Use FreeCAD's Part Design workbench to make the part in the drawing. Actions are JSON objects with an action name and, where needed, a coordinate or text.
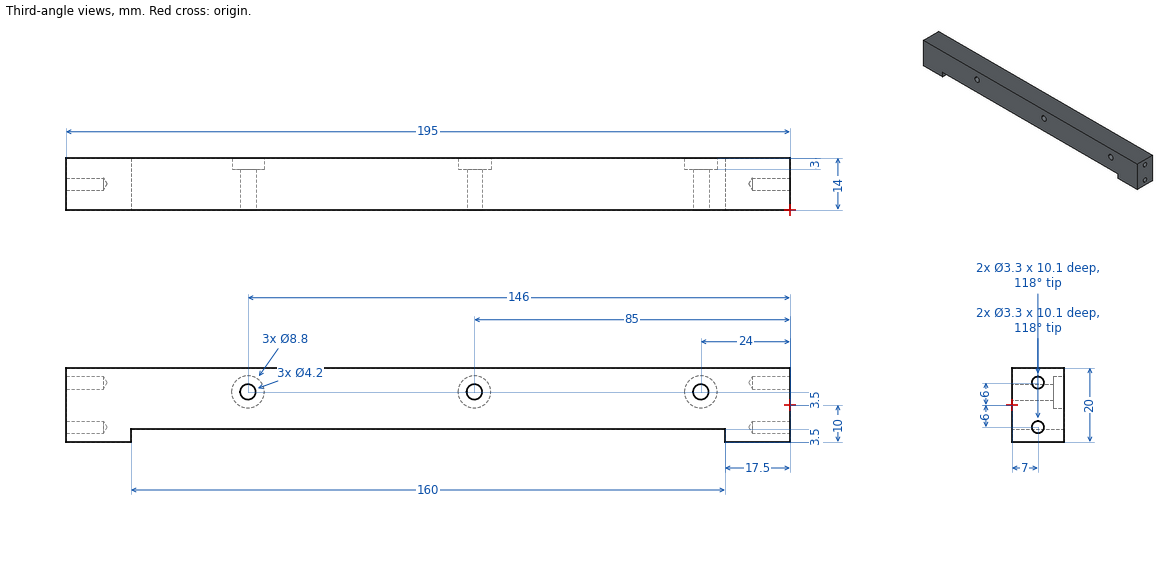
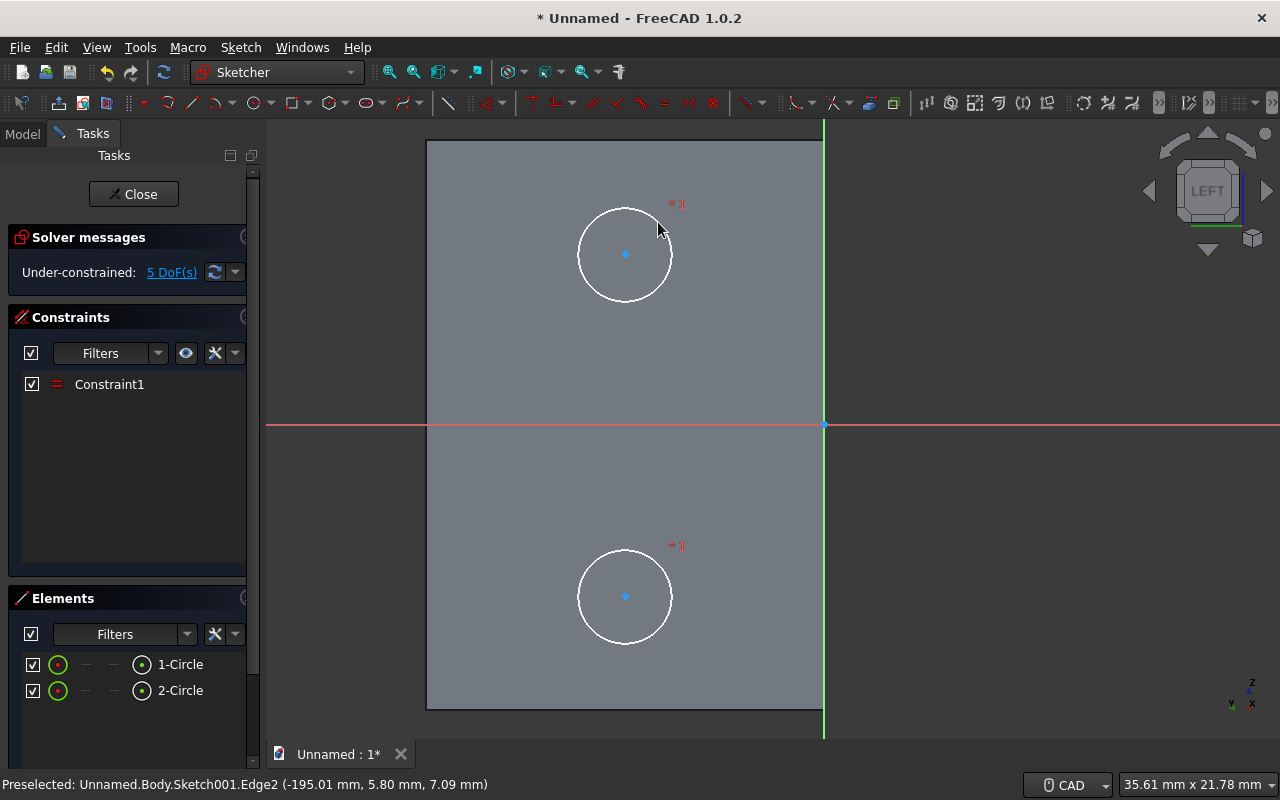
{"action": "left_click", "coordinate": [658, 564]}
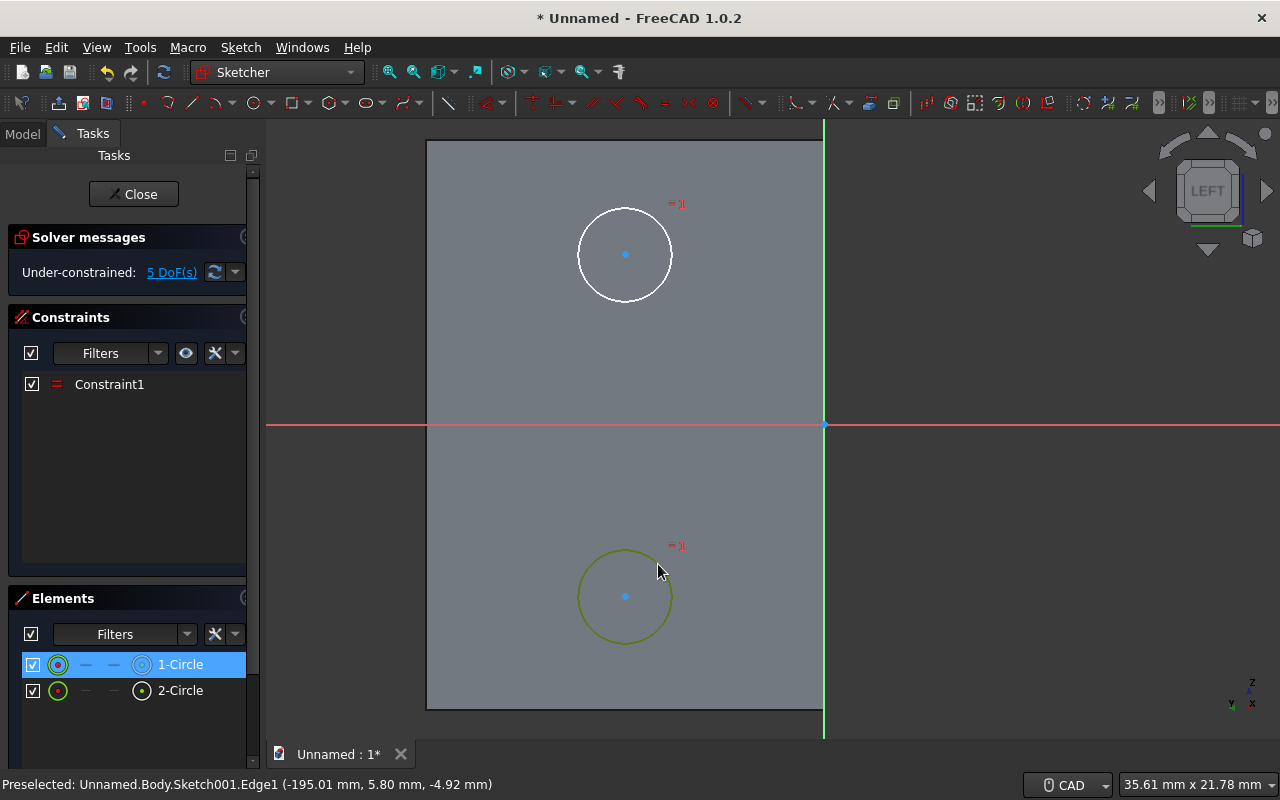
{"action": "key", "text": "k o"}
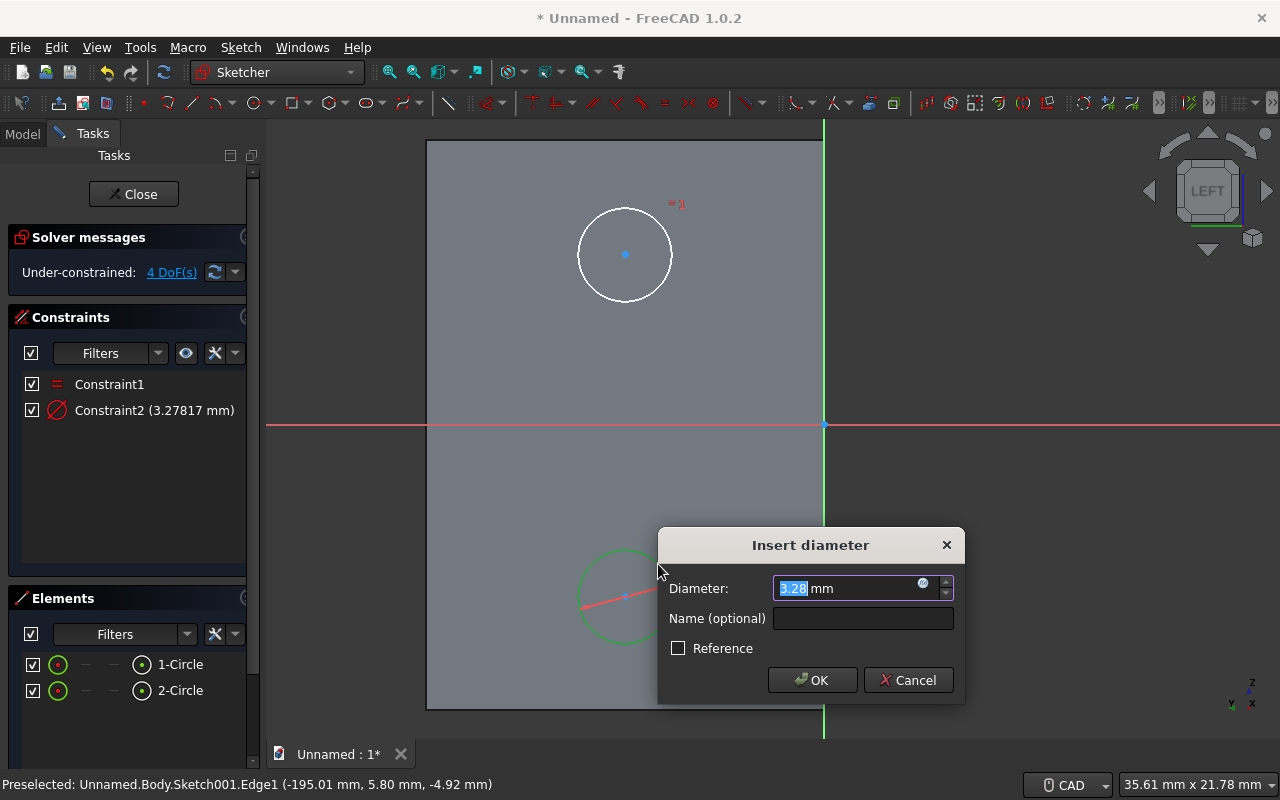
{"action": "type", "text": "3.3"}
{"action": "key", "text": "Return"}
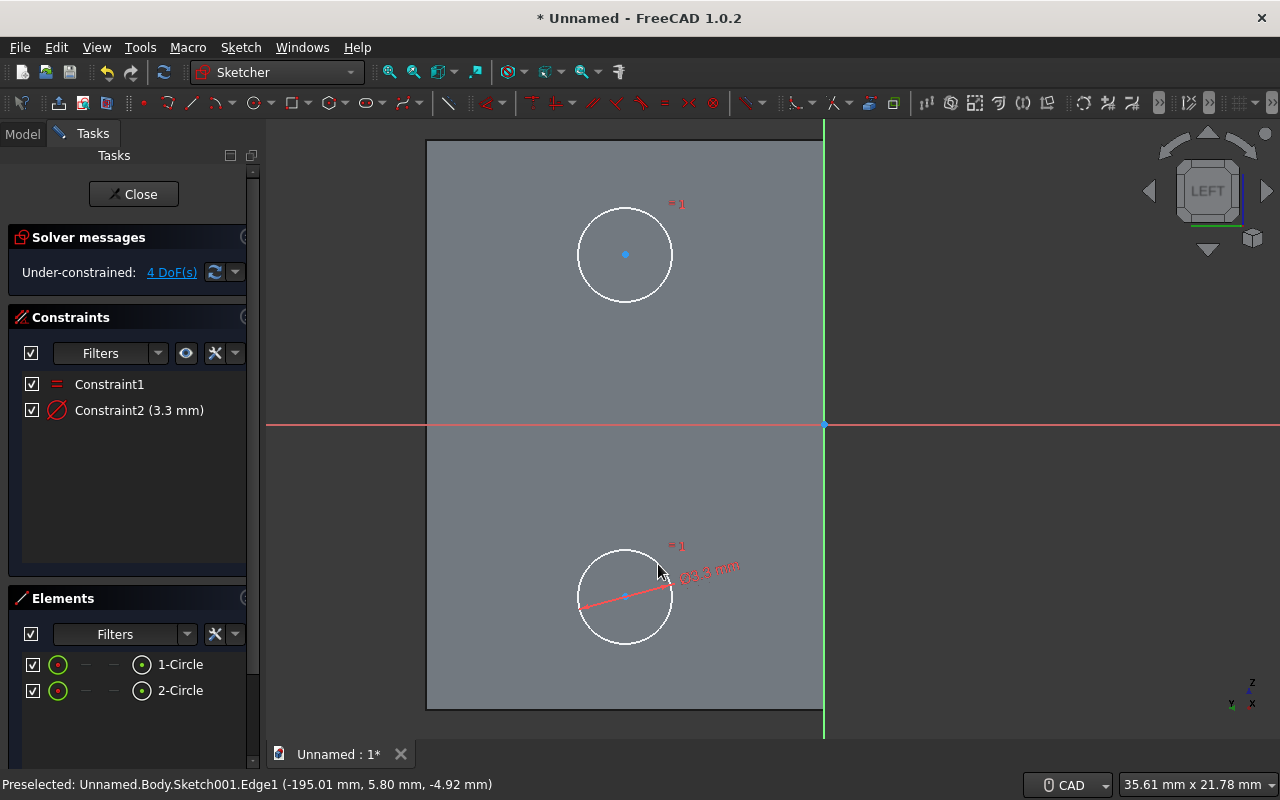
{"action": "left_click", "coordinate": [625, 597]}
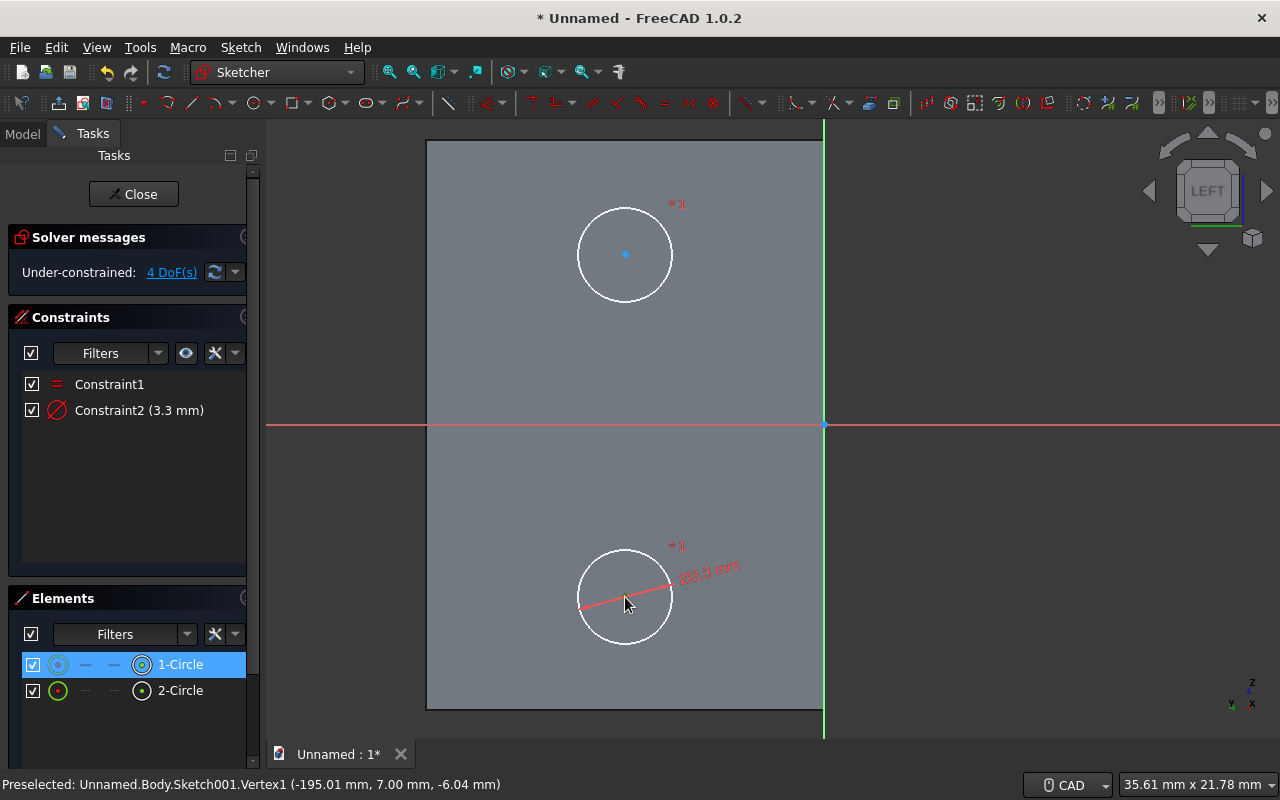
{"action": "key", "text": "l"}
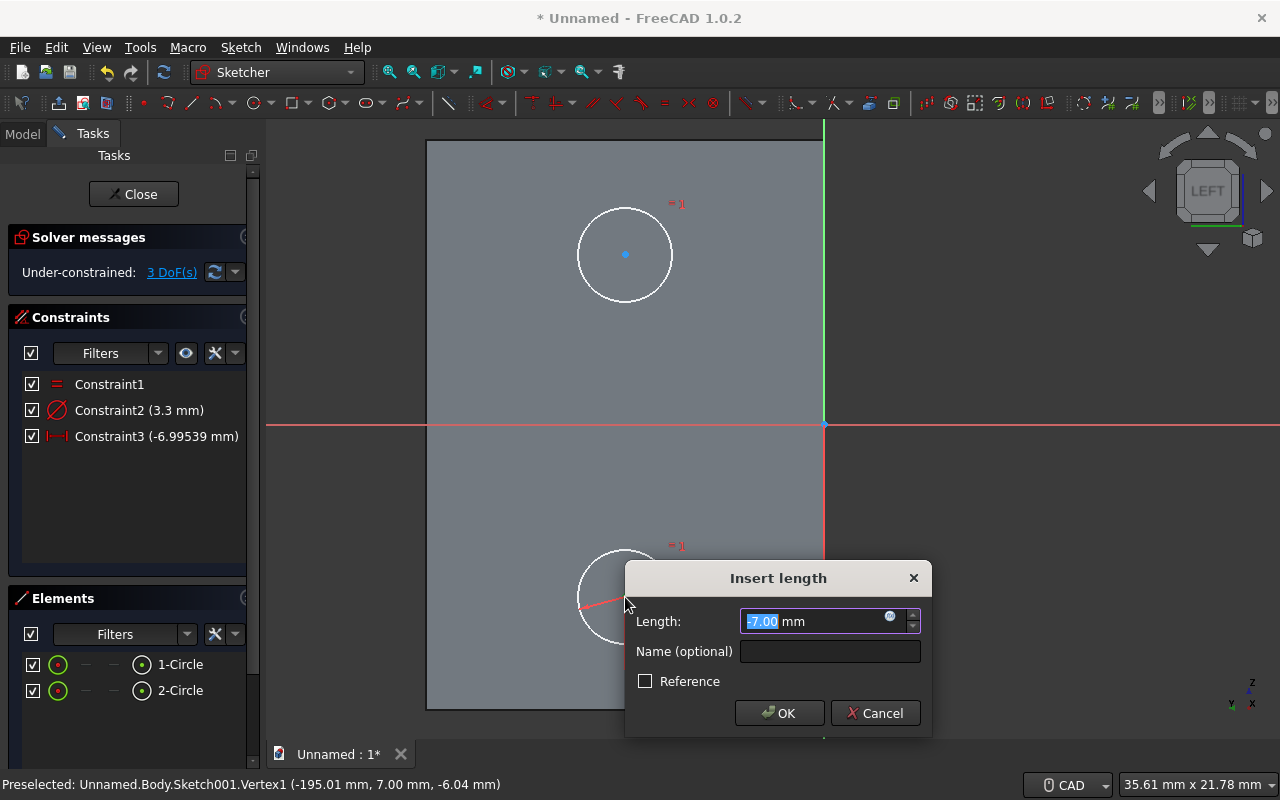
{"action": "type", "text": "-7"}
{"action": "key", "text": "Return"}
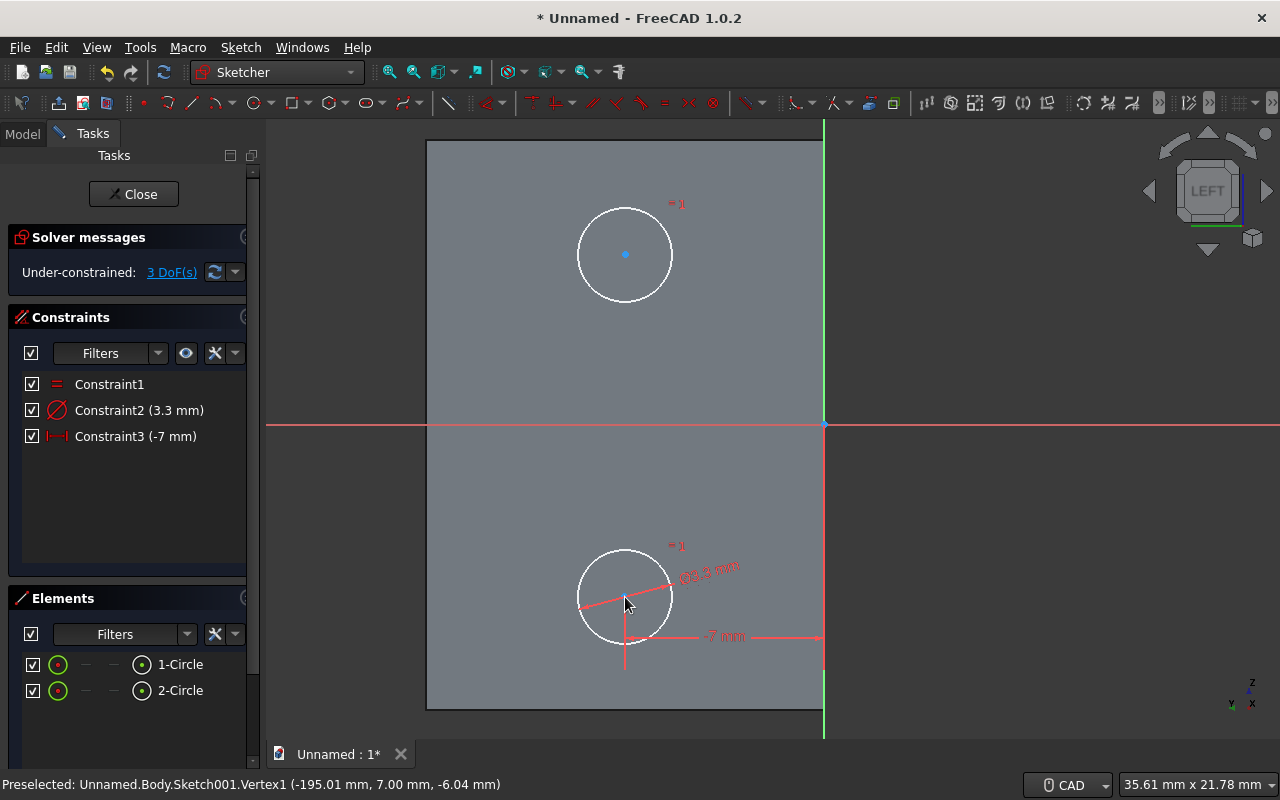
{"action": "left_click", "coordinate": [625, 597]}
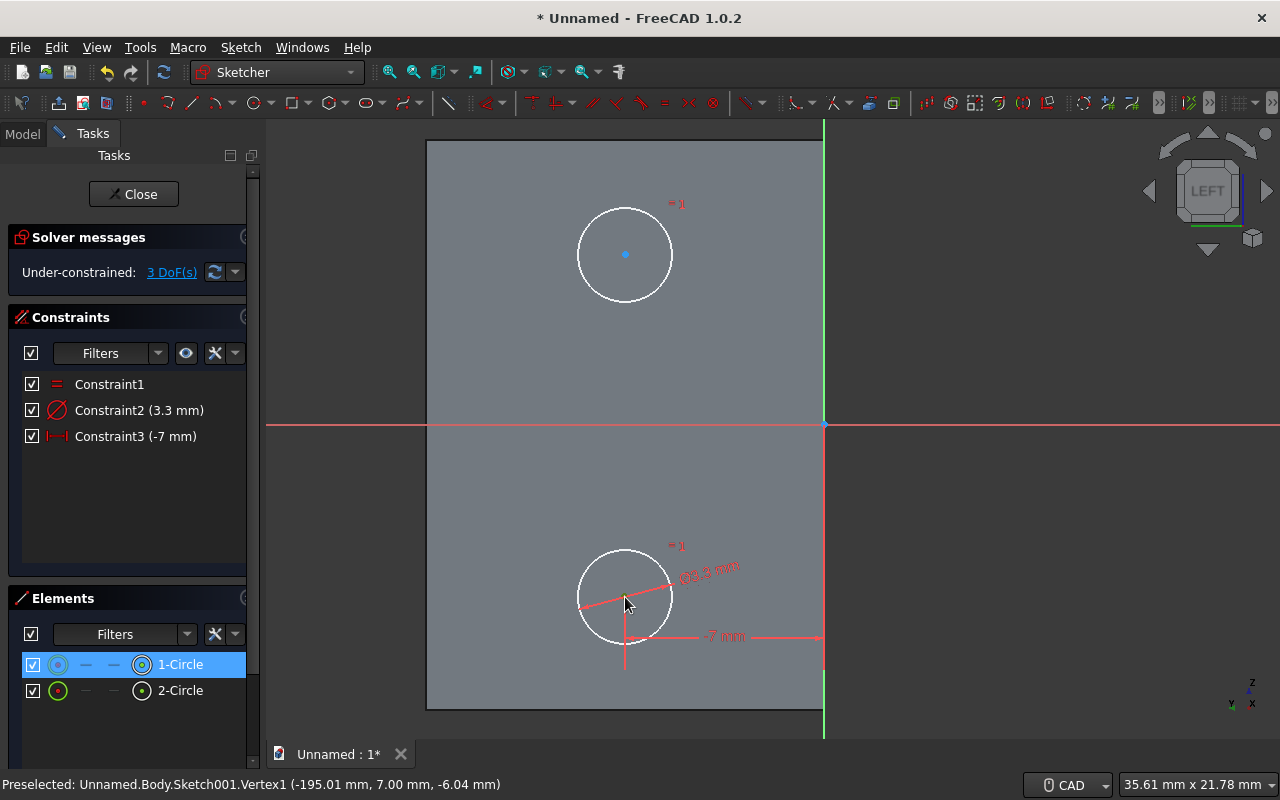
{"action": "left_click", "coordinate": [504, 104]}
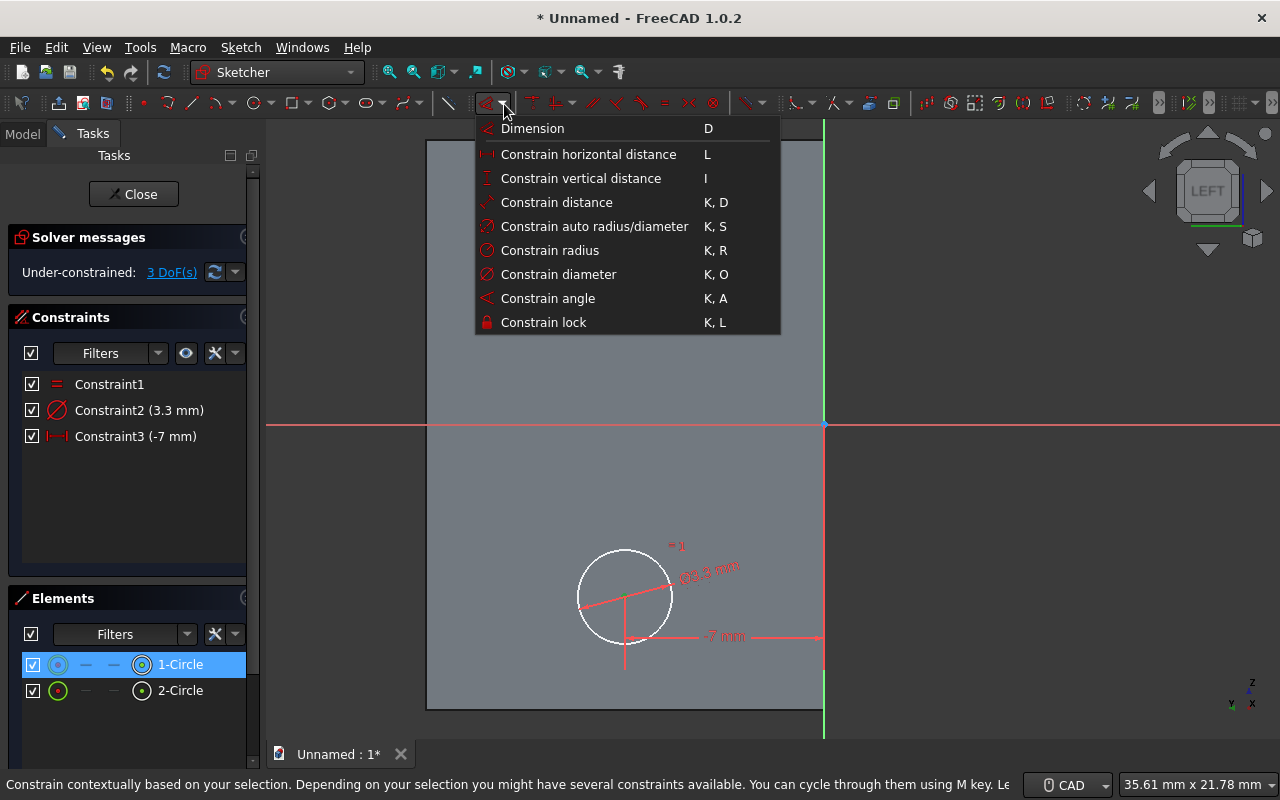
{"action": "left_click", "coordinate": [628, 178]}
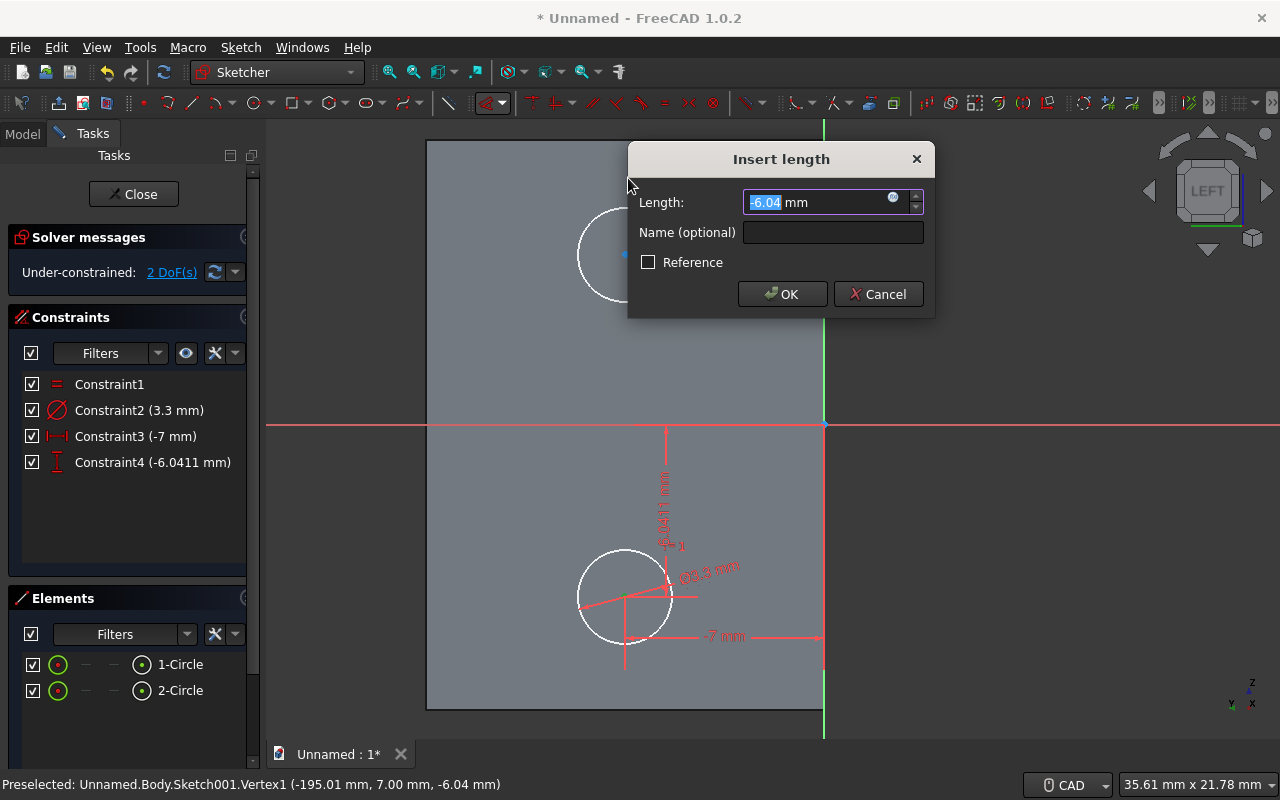
{"action": "type", "text": "-6"}
{"action": "key", "text": "Return"}